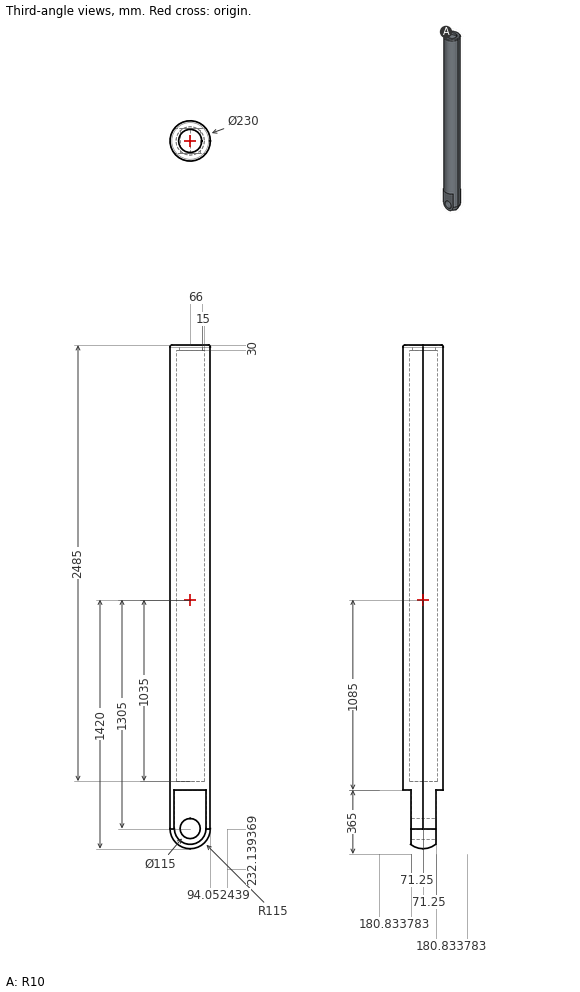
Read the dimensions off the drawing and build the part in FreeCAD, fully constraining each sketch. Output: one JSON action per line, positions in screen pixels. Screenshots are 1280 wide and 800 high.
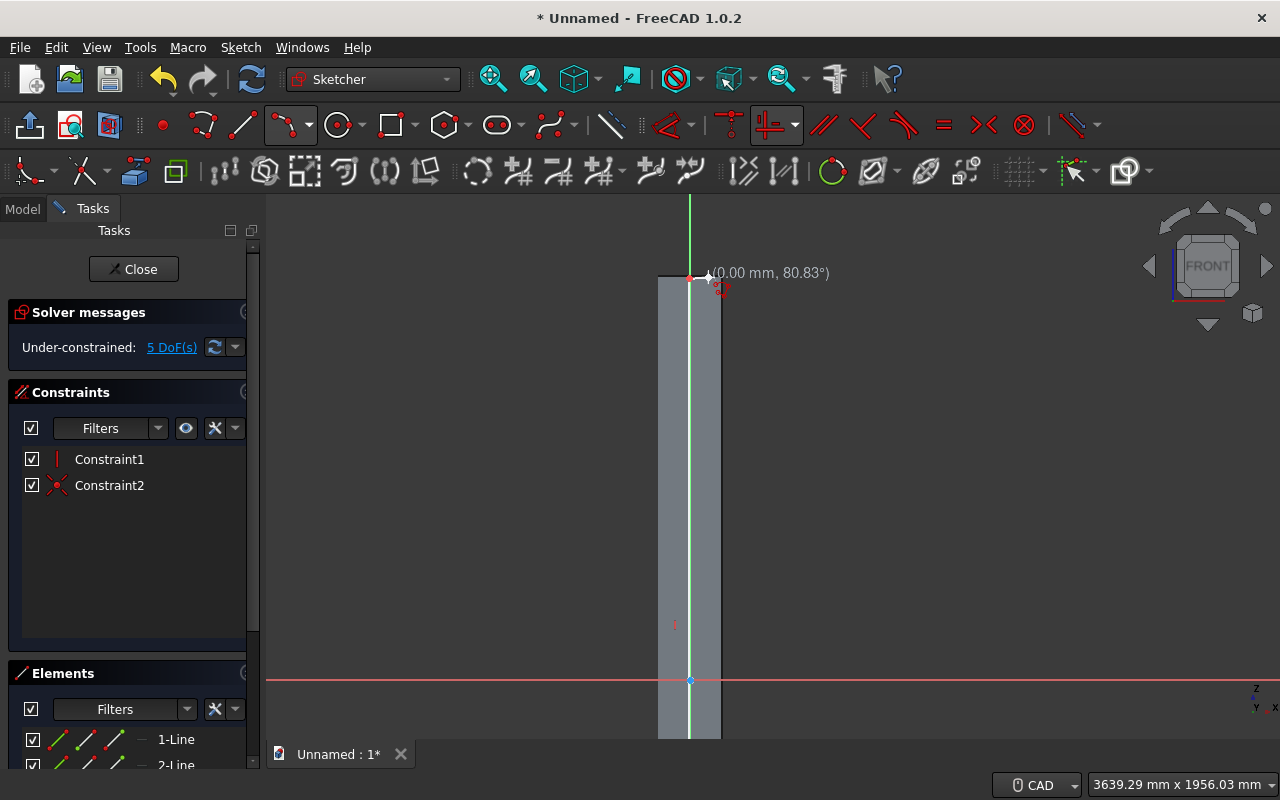
{"action": "scroll", "coordinate": [708, 285], "scroll_direction": "up", "scroll_amount": 4}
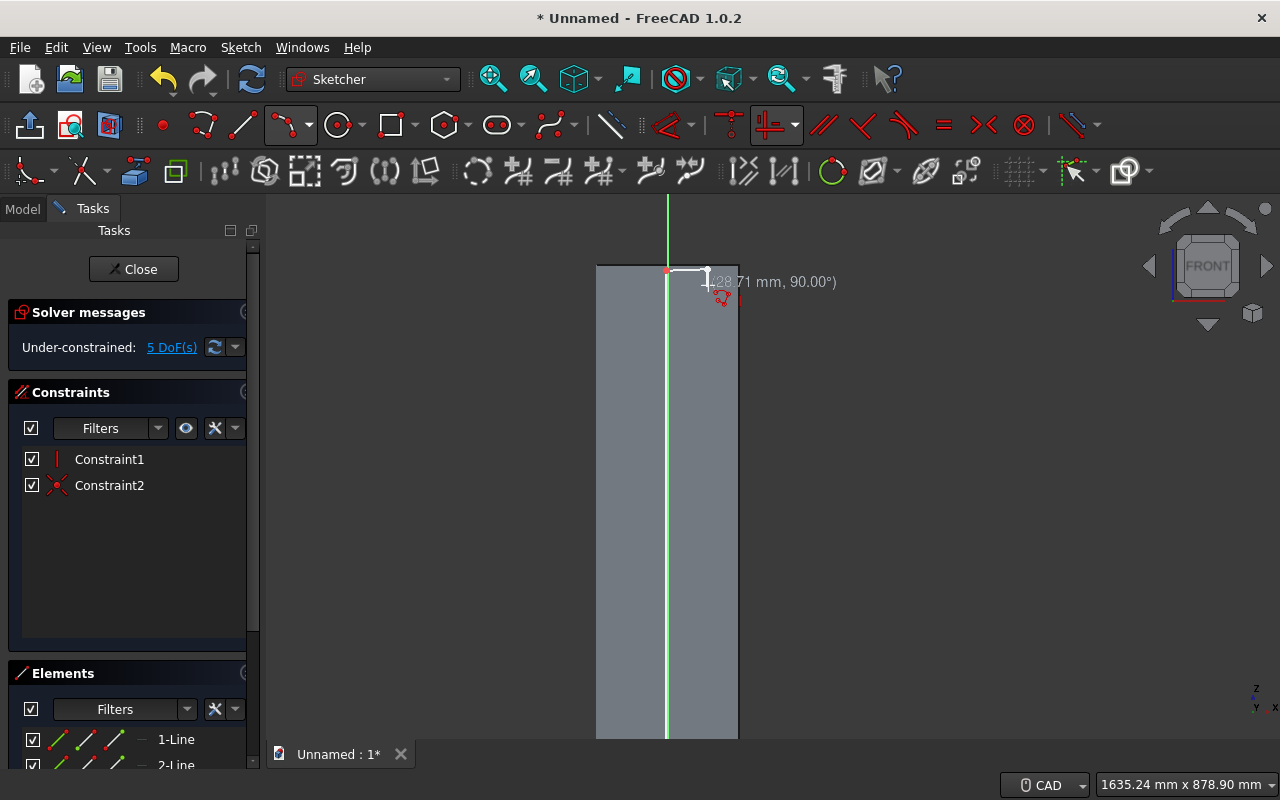
{"action": "left_click", "coordinate": [707, 284]}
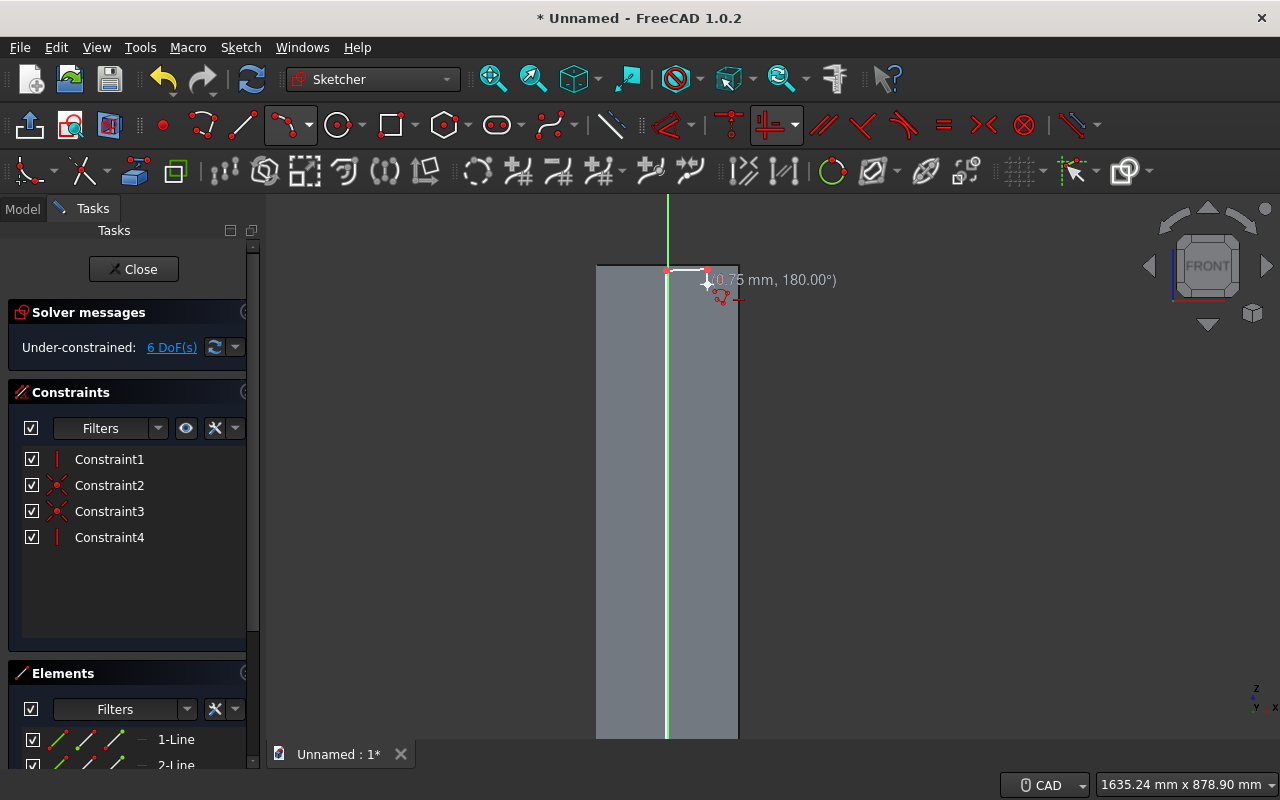
{"action": "scroll", "coordinate": [718, 284], "scroll_direction": "up", "scroll_amount": 3}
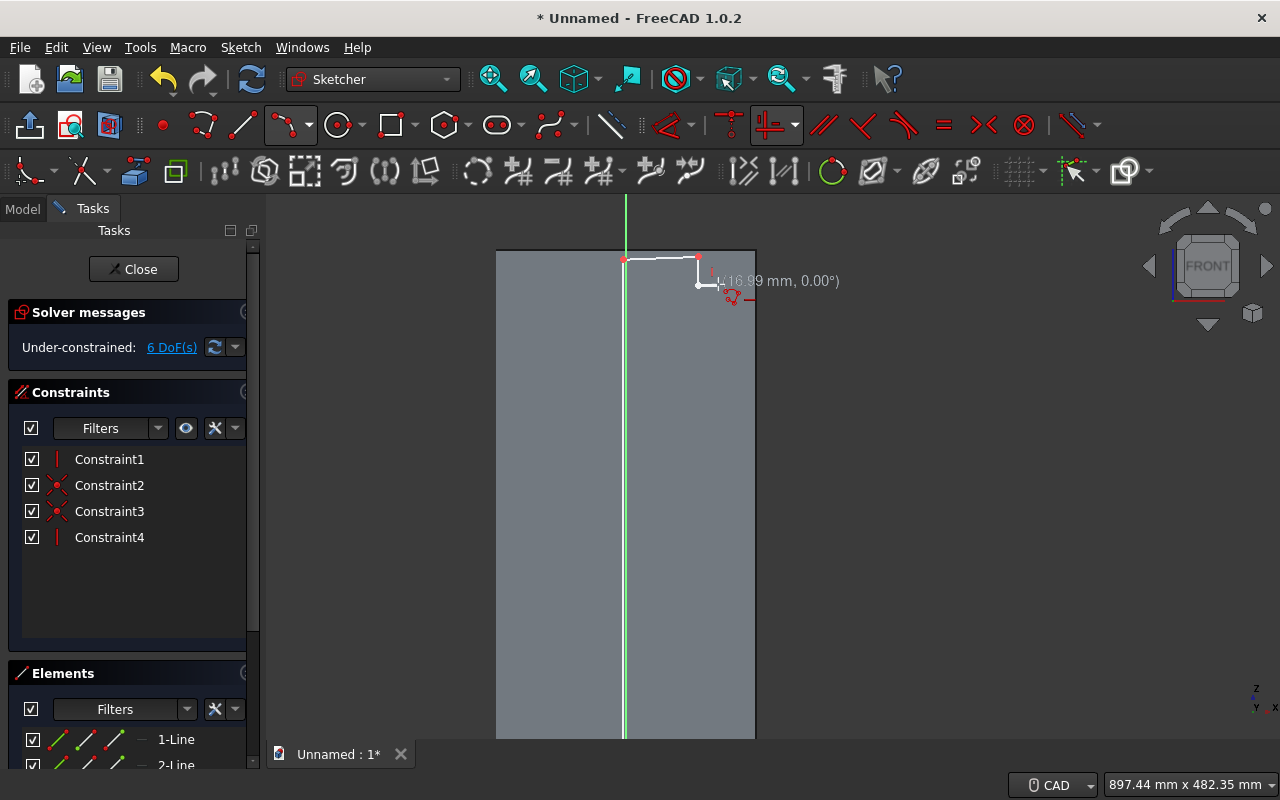
{"action": "left_click", "coordinate": [717, 284]}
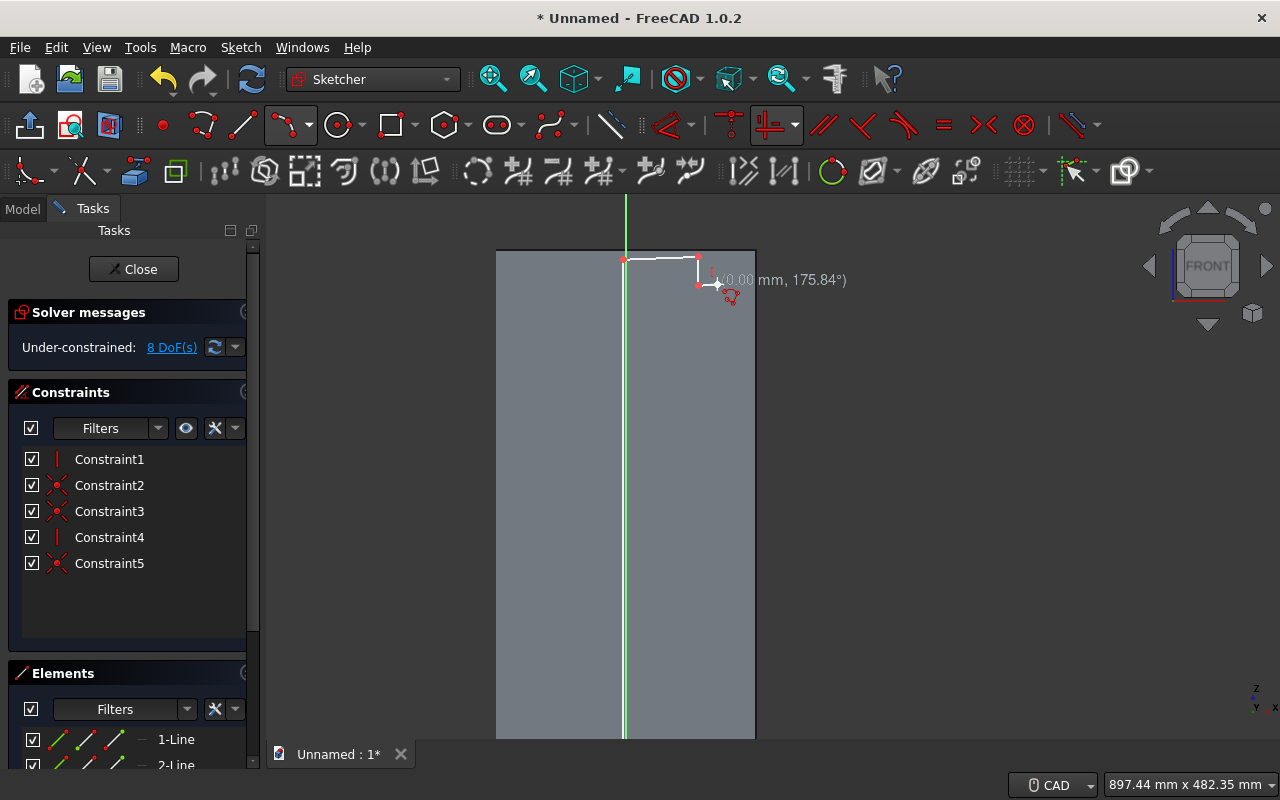
{"action": "scroll", "coordinate": [710, 281], "scroll_direction": "down", "scroll_amount": 10}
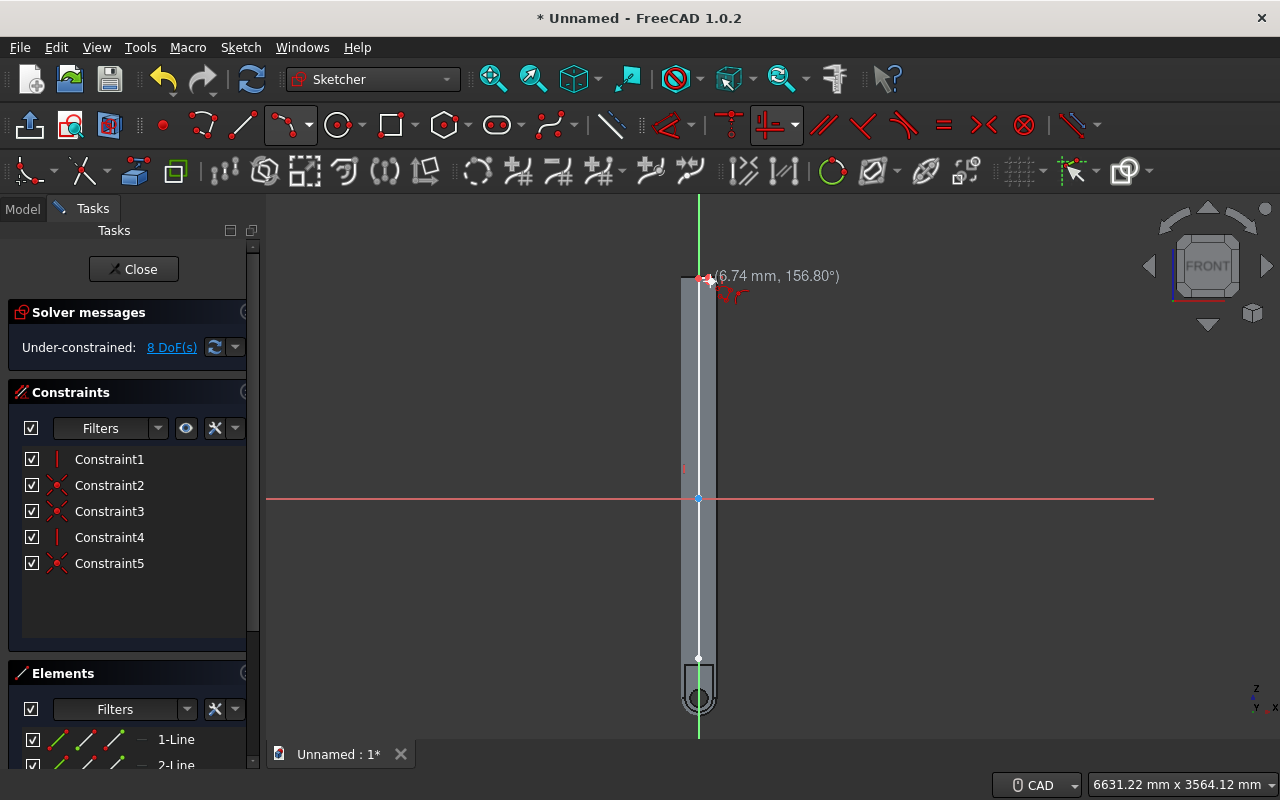
{"action": "scroll", "coordinate": [711, 657], "scroll_direction": "up", "scroll_amount": 2}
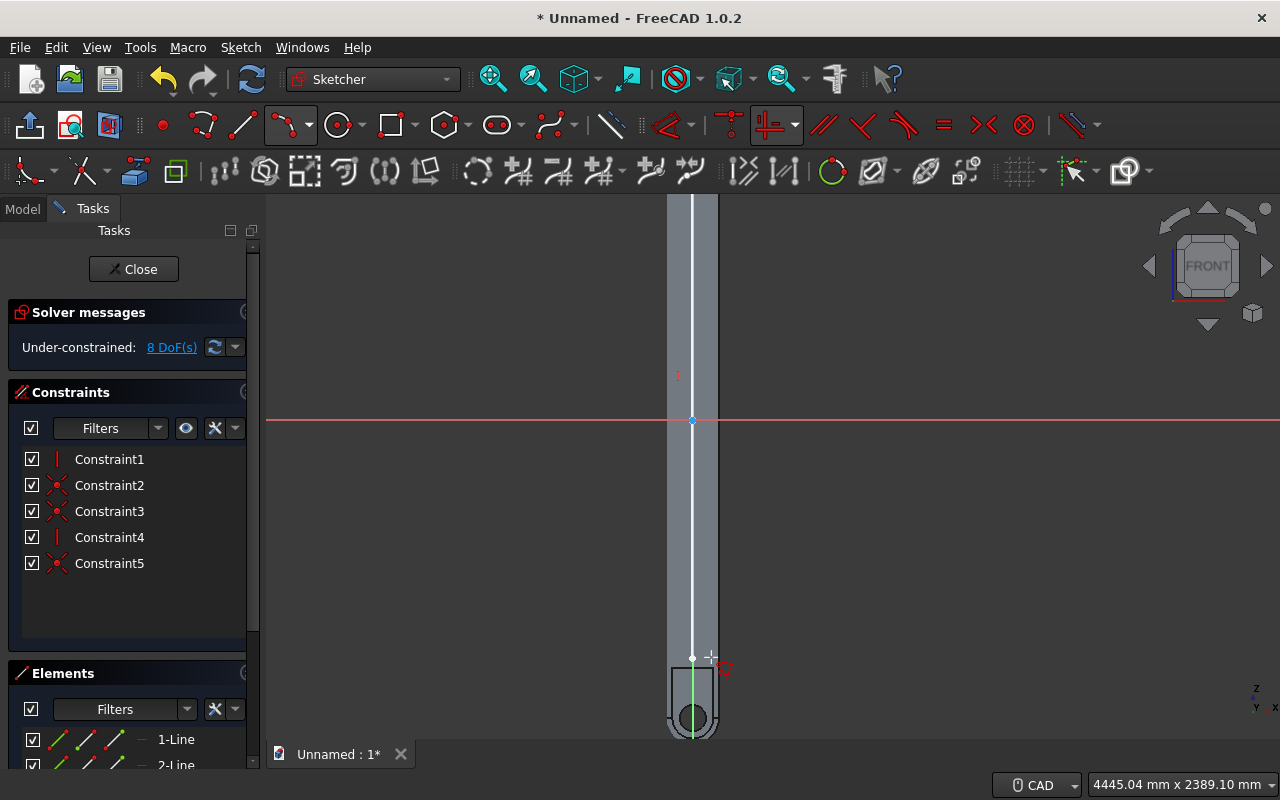
{"action": "left_click", "coordinate": [711, 656]}
{"action": "left_click", "coordinate": [692, 658]}
{"action": "key", "text": "Escape"}
{"action": "key", "text": "Escape"}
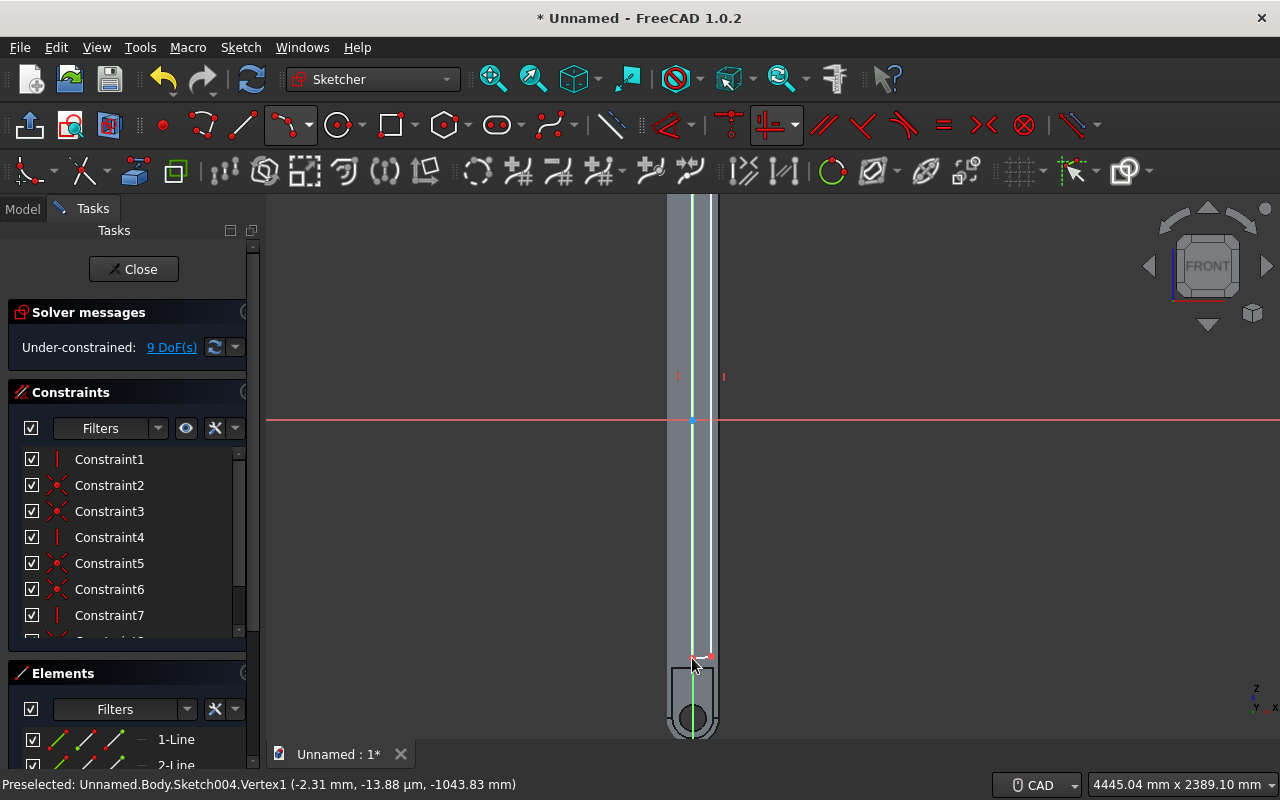
{"action": "scroll", "coordinate": [709, 657], "scroll_direction": "down", "scroll_amount": 2}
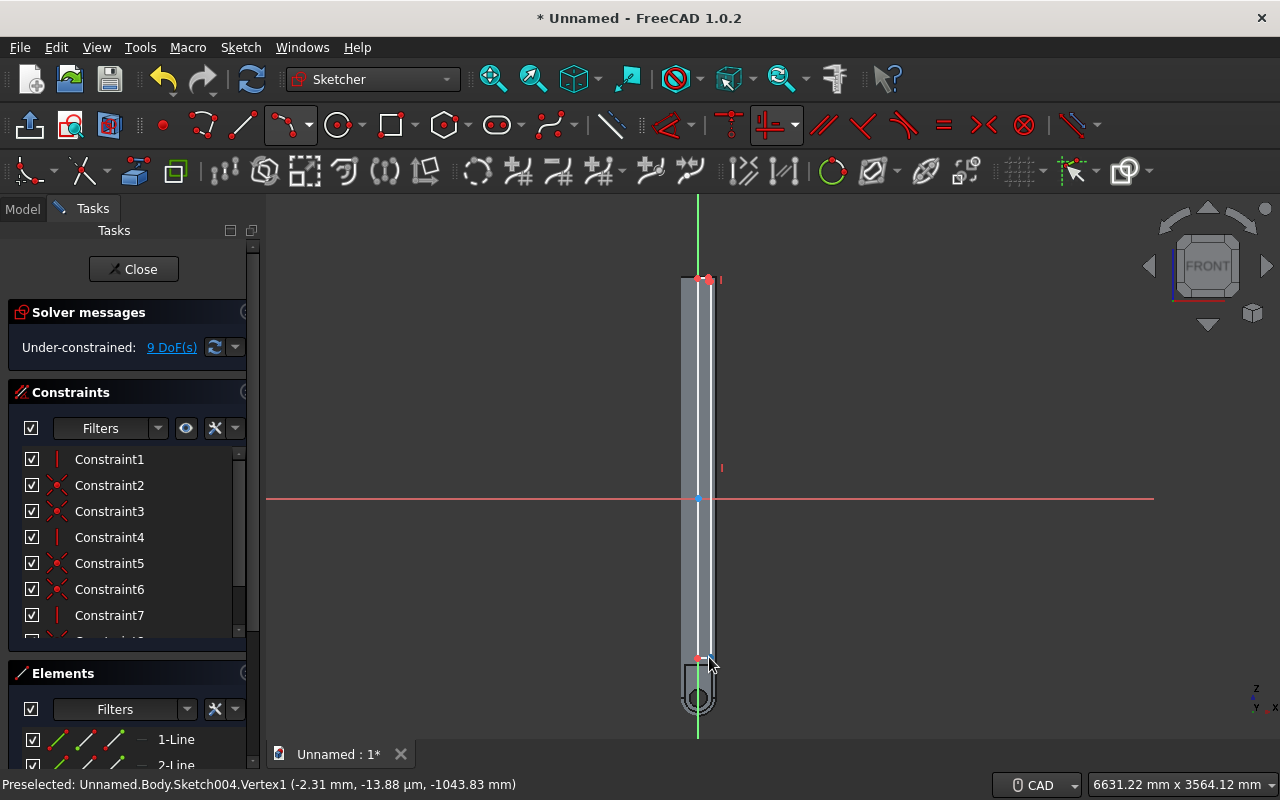
{"action": "scroll", "coordinate": [703, 278], "scroll_direction": "up", "scroll_amount": 6}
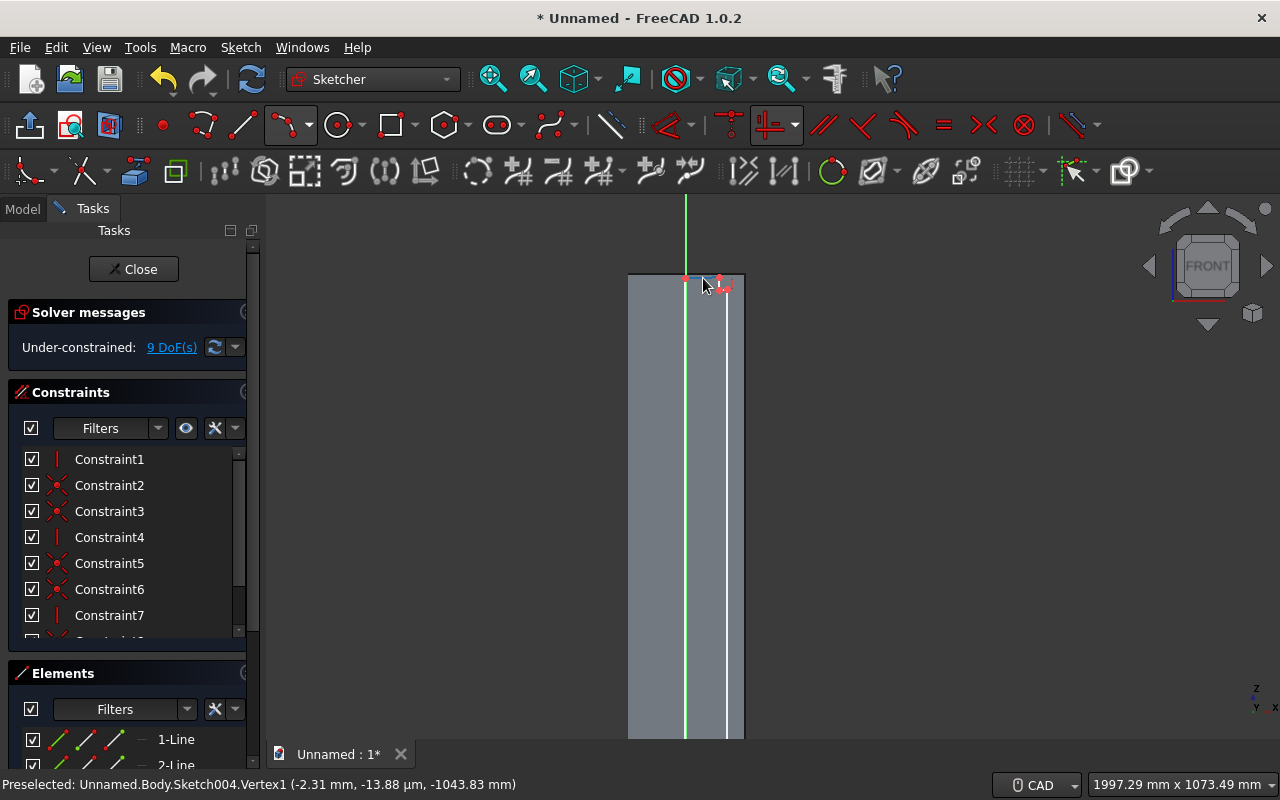
{"action": "left_click", "coordinate": [702, 278]}